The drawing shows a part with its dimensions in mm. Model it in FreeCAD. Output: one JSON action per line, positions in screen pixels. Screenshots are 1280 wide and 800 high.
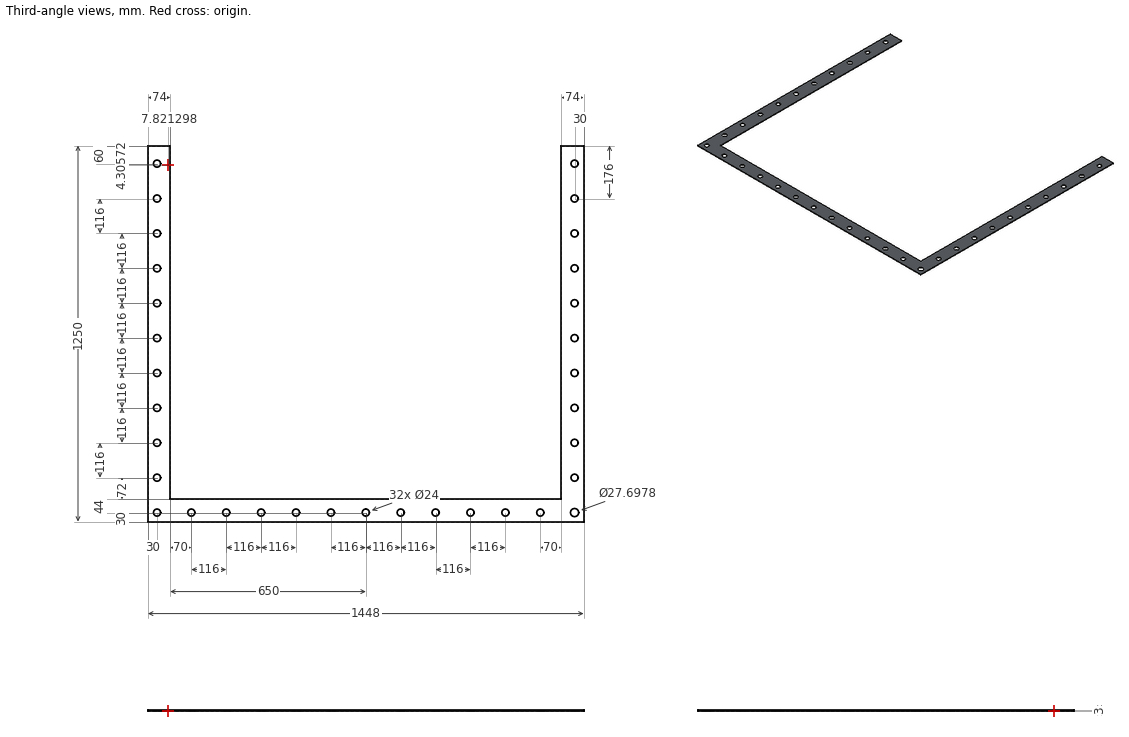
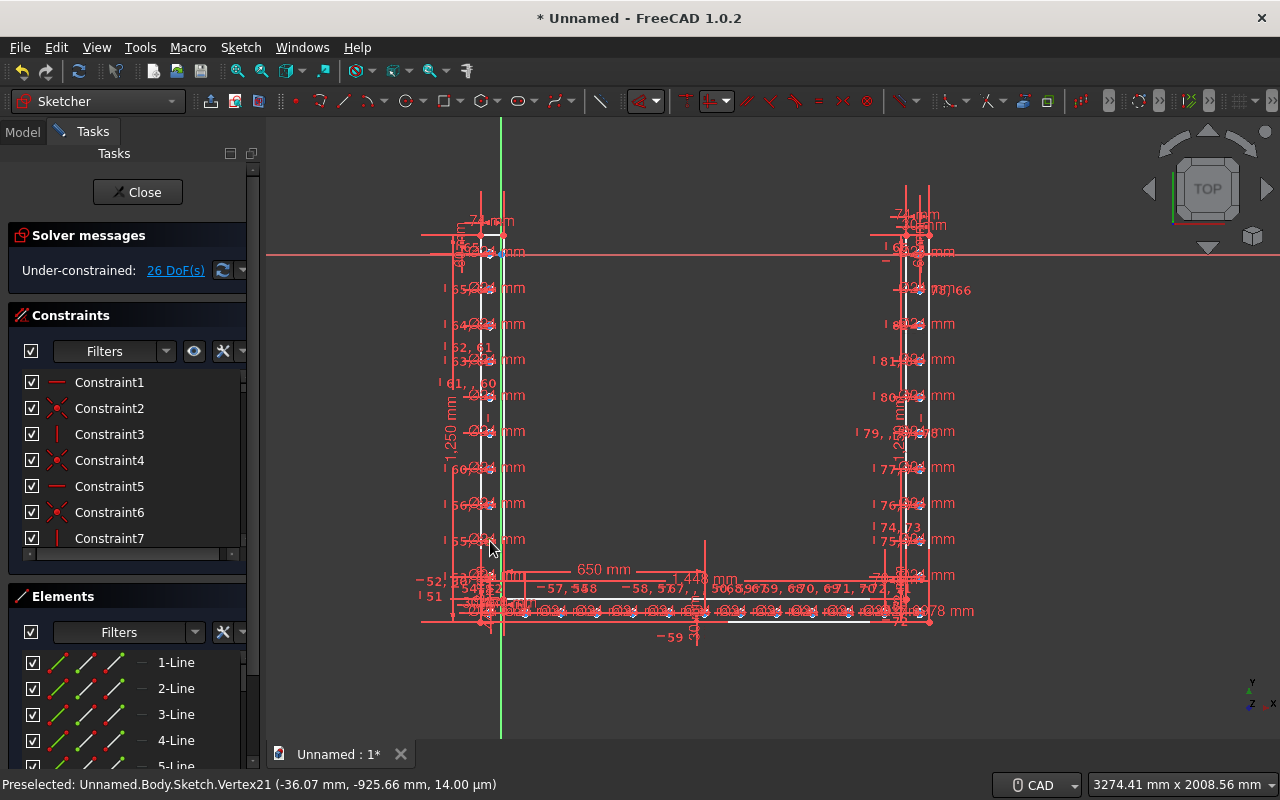
{"action": "key", "text": "i"}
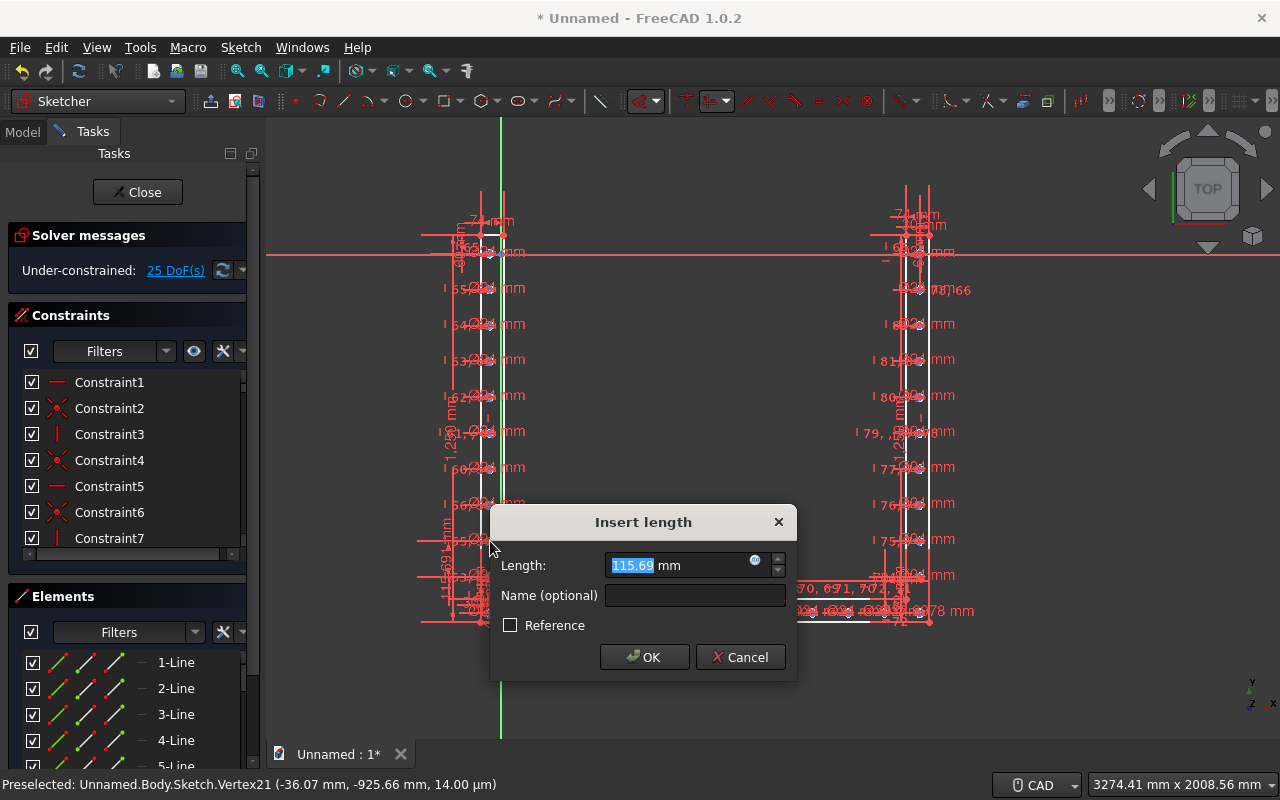
{"action": "type", "text": "116"}
{"action": "key", "text": "Return"}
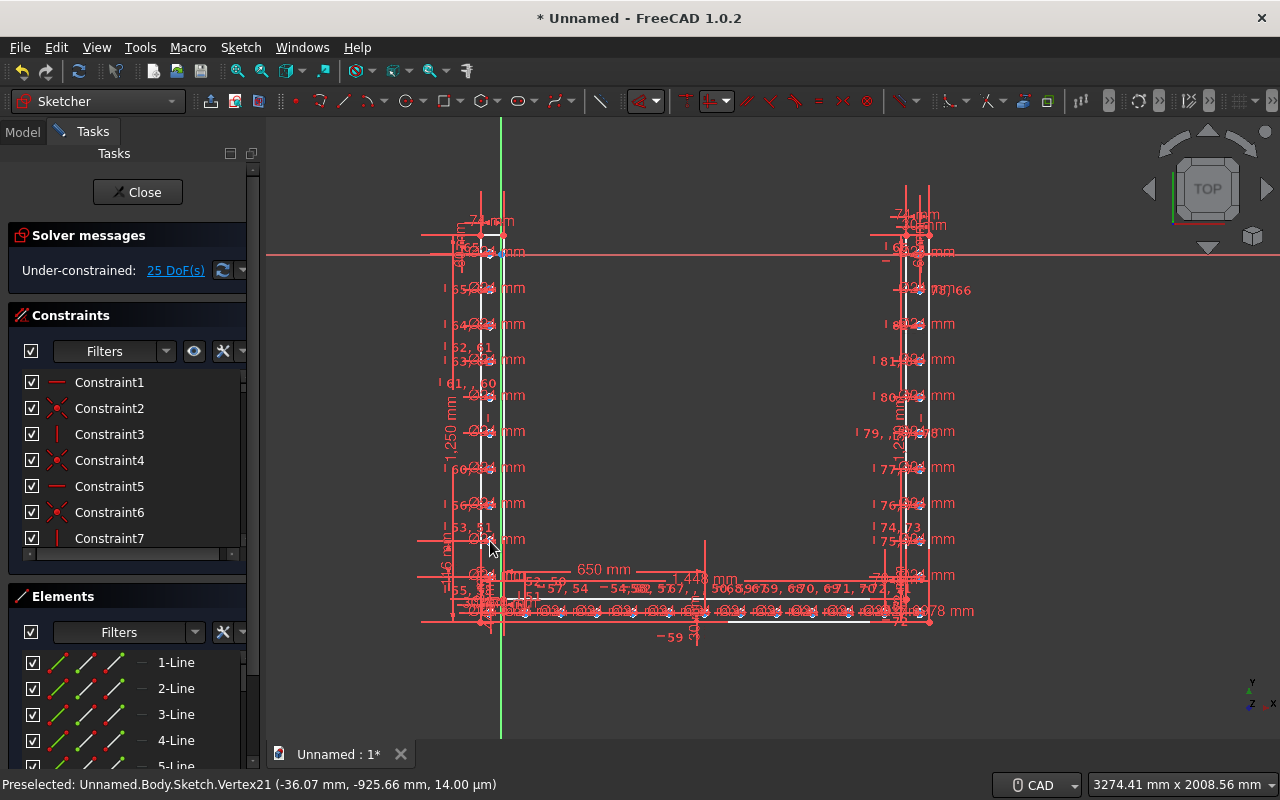
{"action": "left_click", "coordinate": [525, 613]}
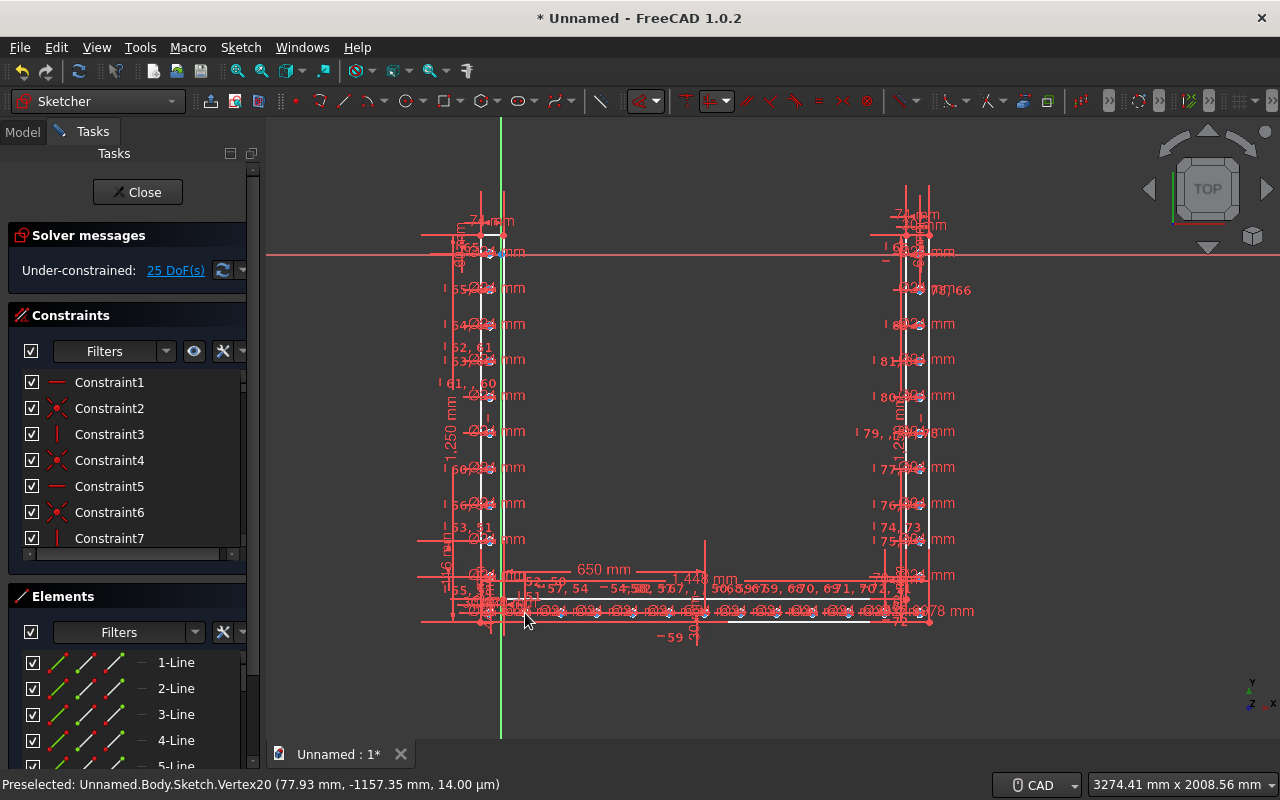
{"action": "left_click", "coordinate": [561, 613]}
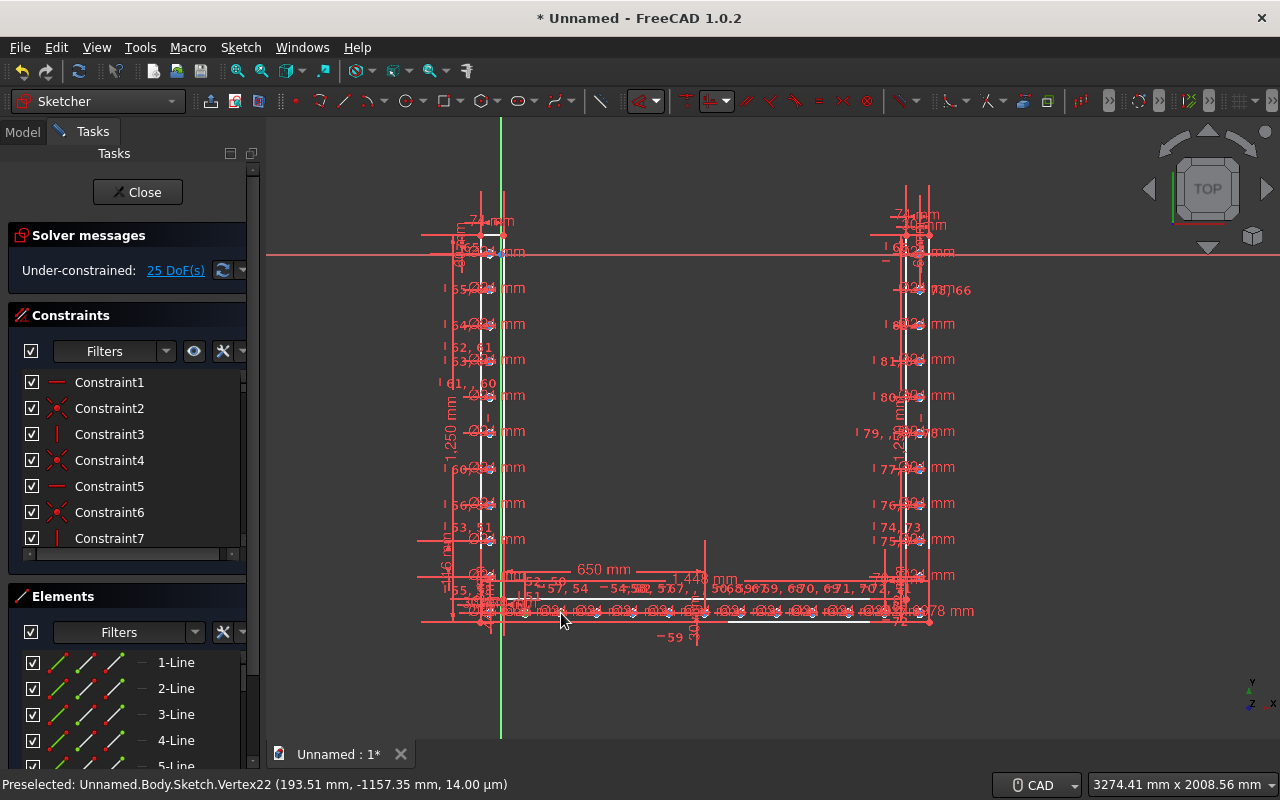
{"action": "left_click", "coordinate": [658, 102]}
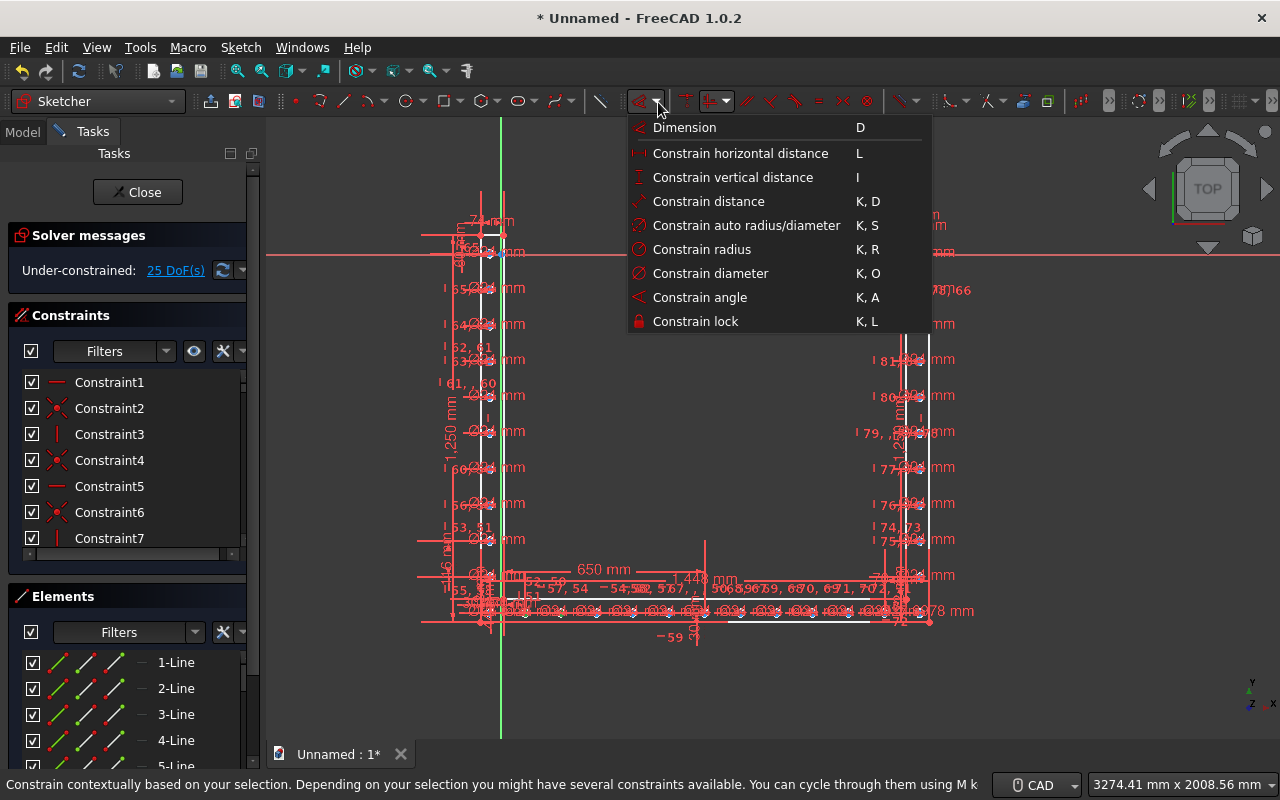
{"action": "left_click", "coordinate": [780, 153]}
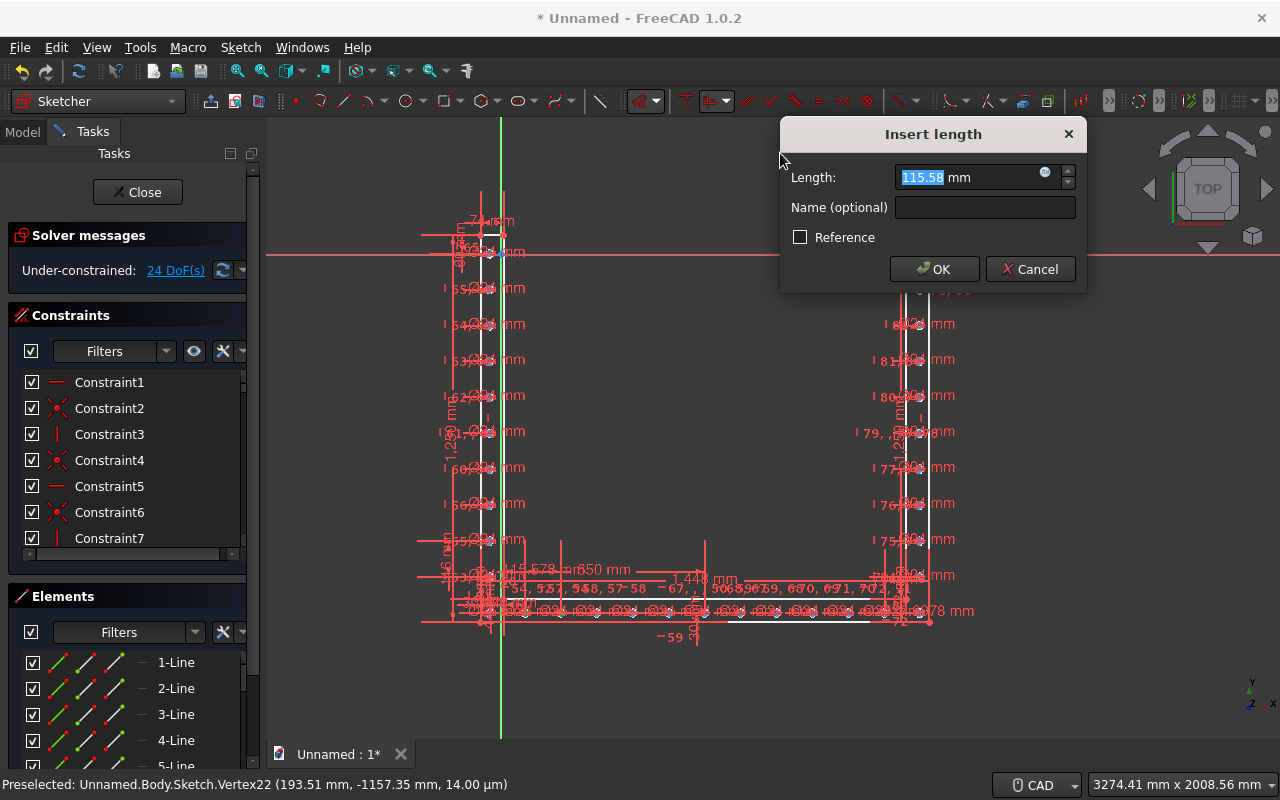
{"action": "type", "text": "116"}
{"action": "key", "text": "Return"}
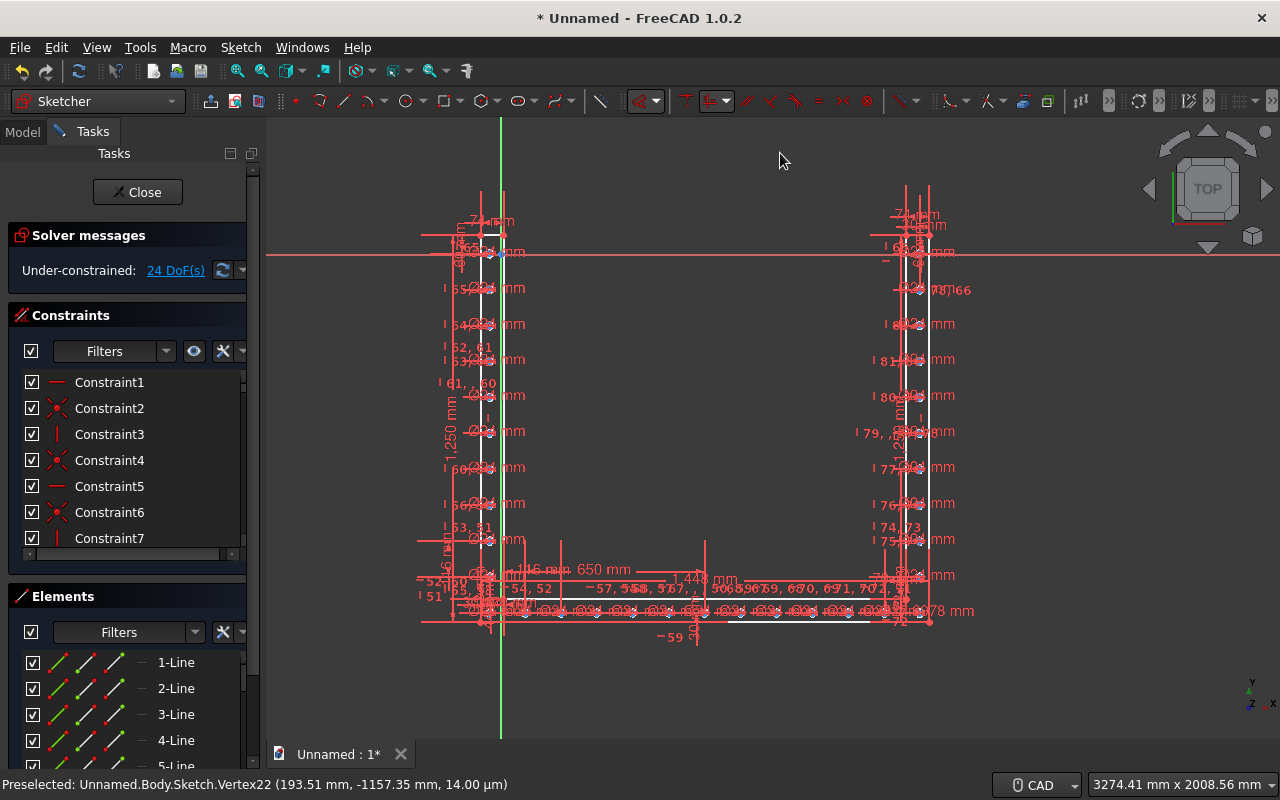
{"action": "left_click", "coordinate": [490, 541]}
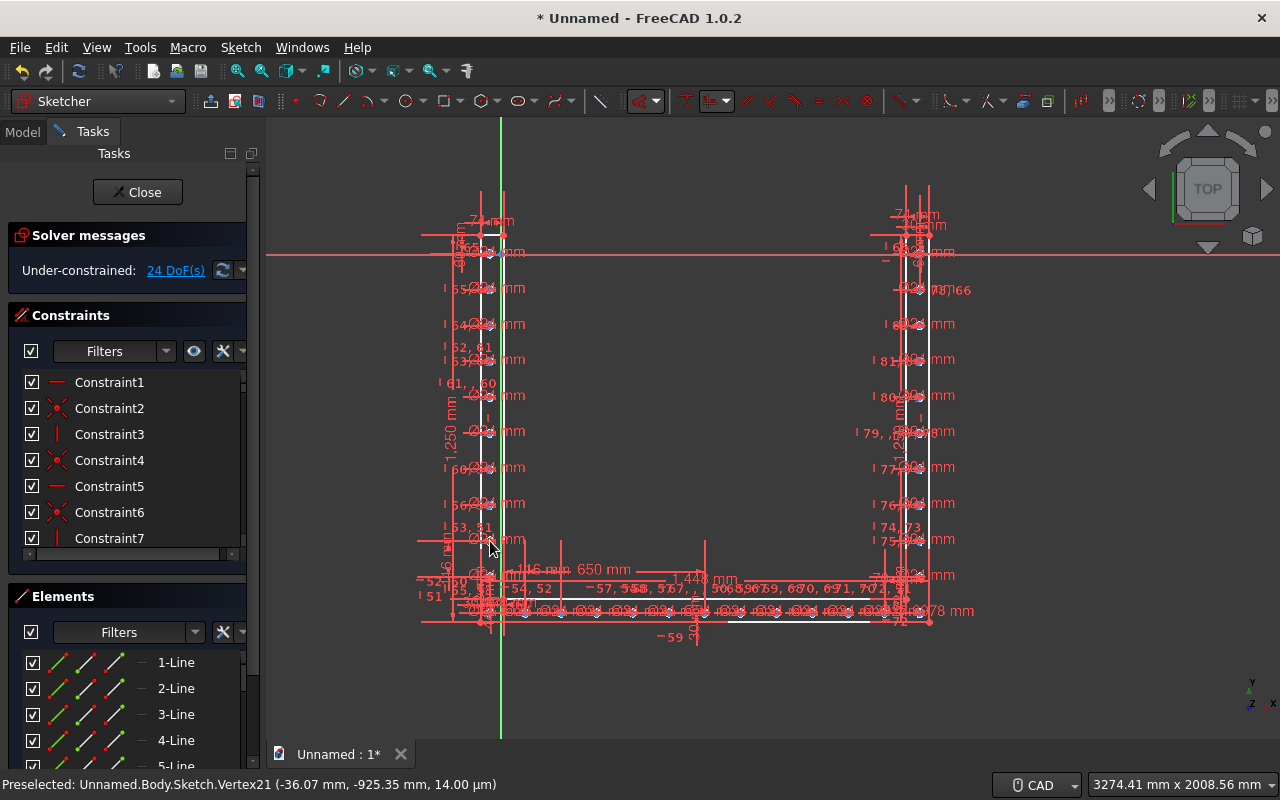
{"action": "left_click", "coordinate": [490, 505]}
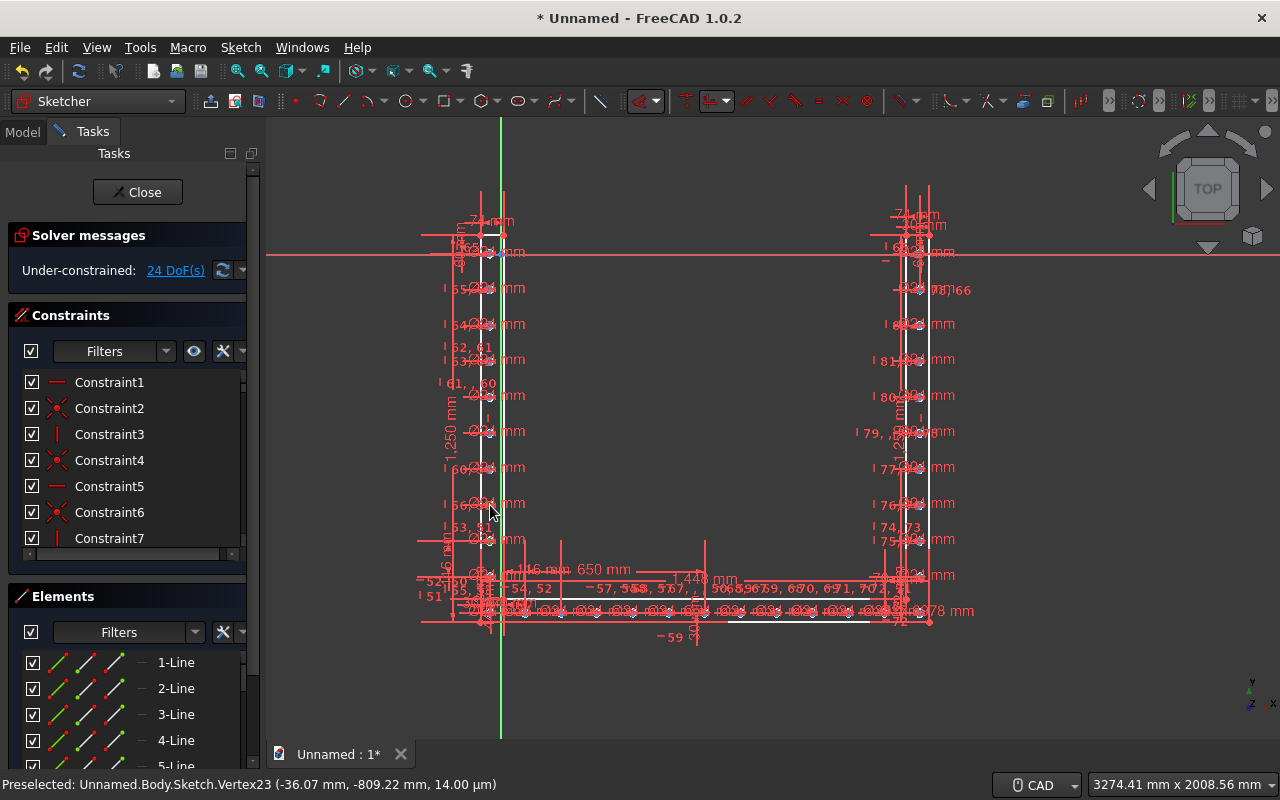
{"action": "key", "text": "i"}